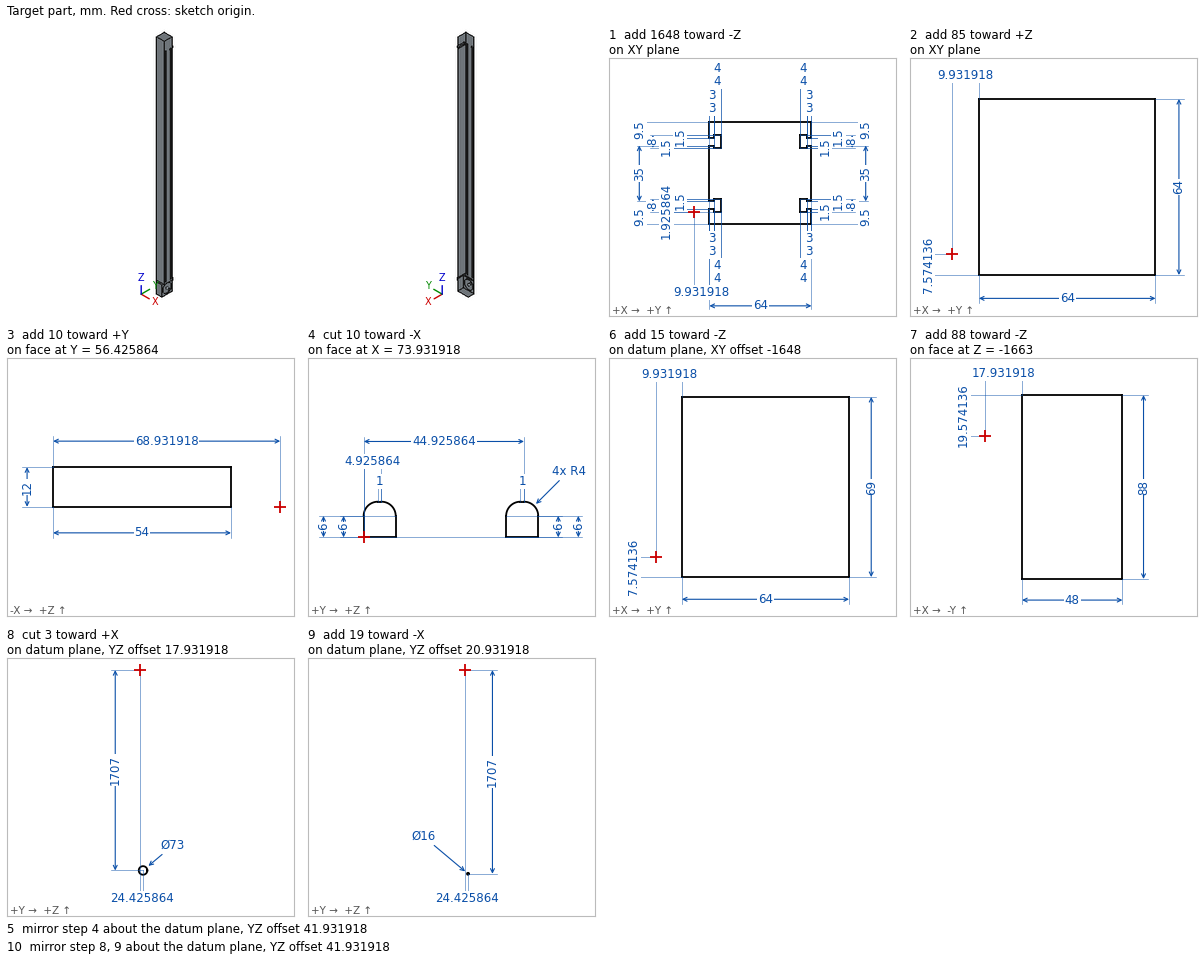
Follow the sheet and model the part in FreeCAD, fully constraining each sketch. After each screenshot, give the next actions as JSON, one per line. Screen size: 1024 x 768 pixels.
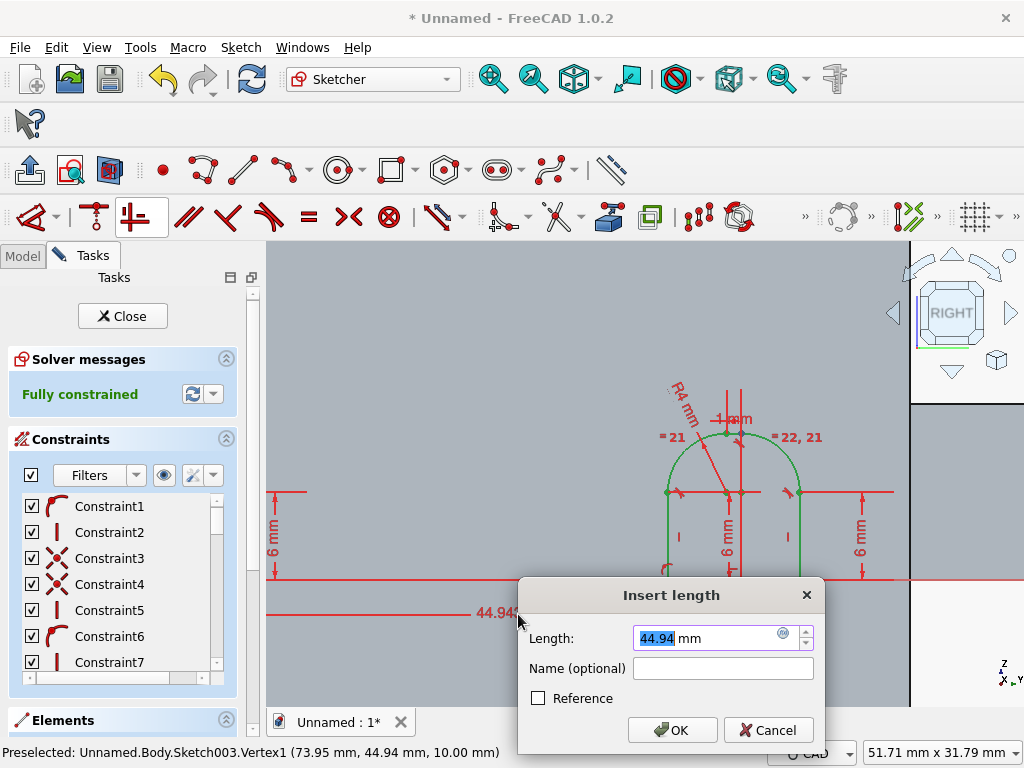
{"action": "type", "text": "44.925864"}
{"action": "key", "text": "Return"}
{"action": "key", "text": "Escape"}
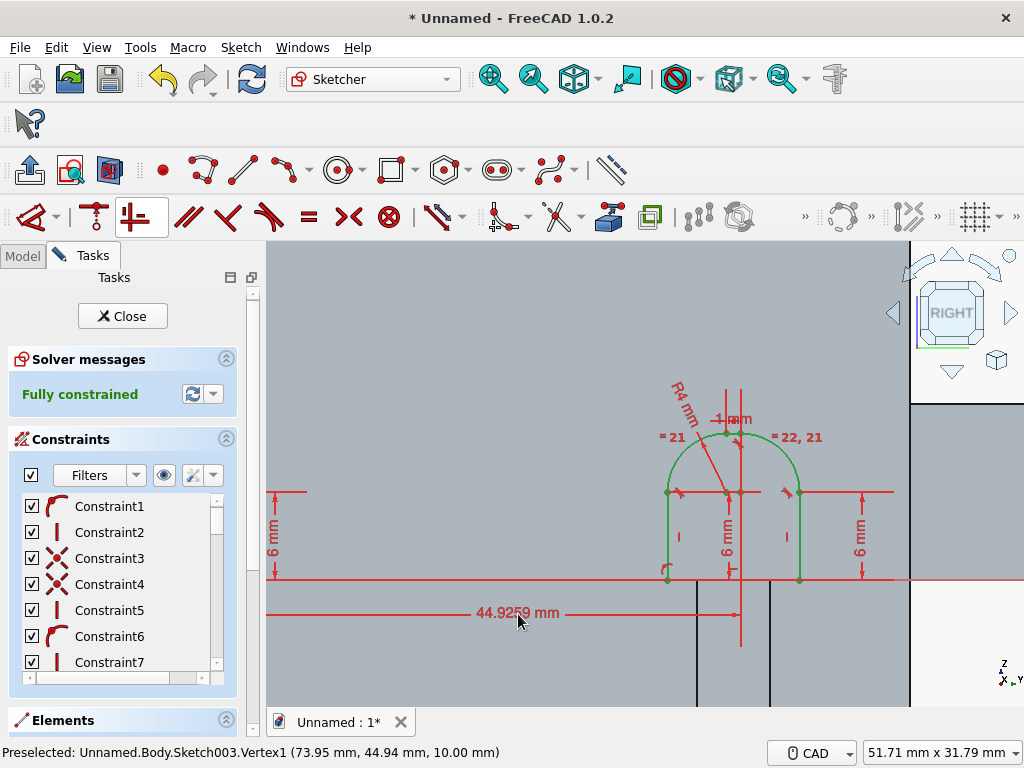
{"action": "left_click", "coordinate": [123, 316]}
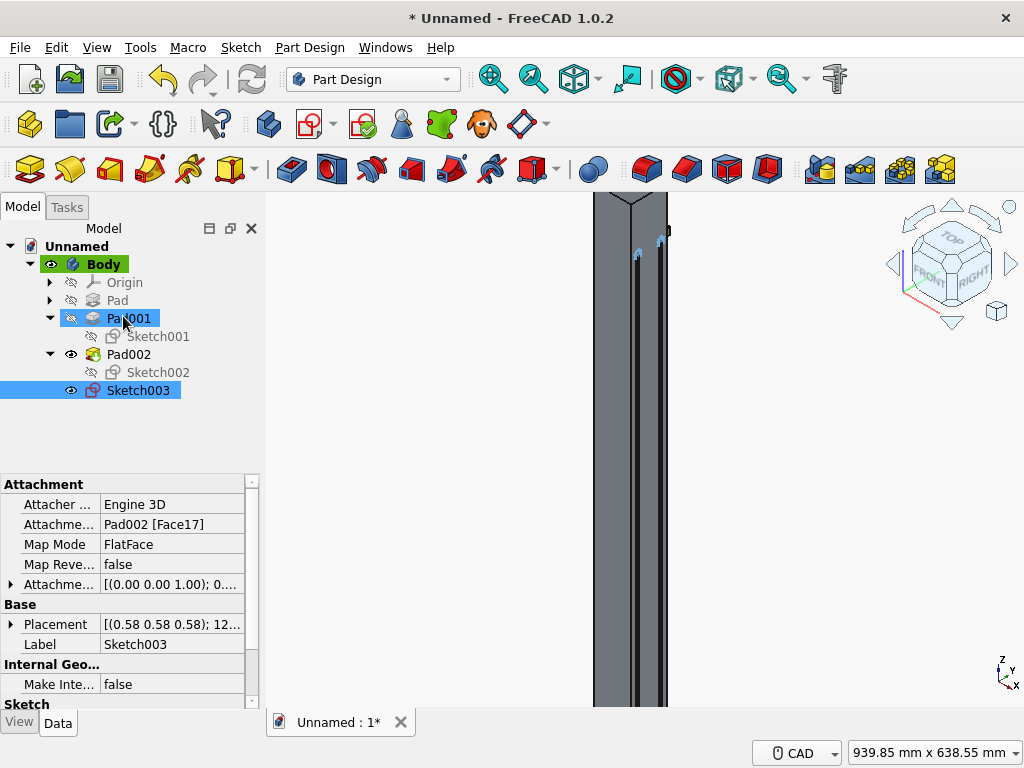
{"action": "left_click", "coordinate": [292, 170]}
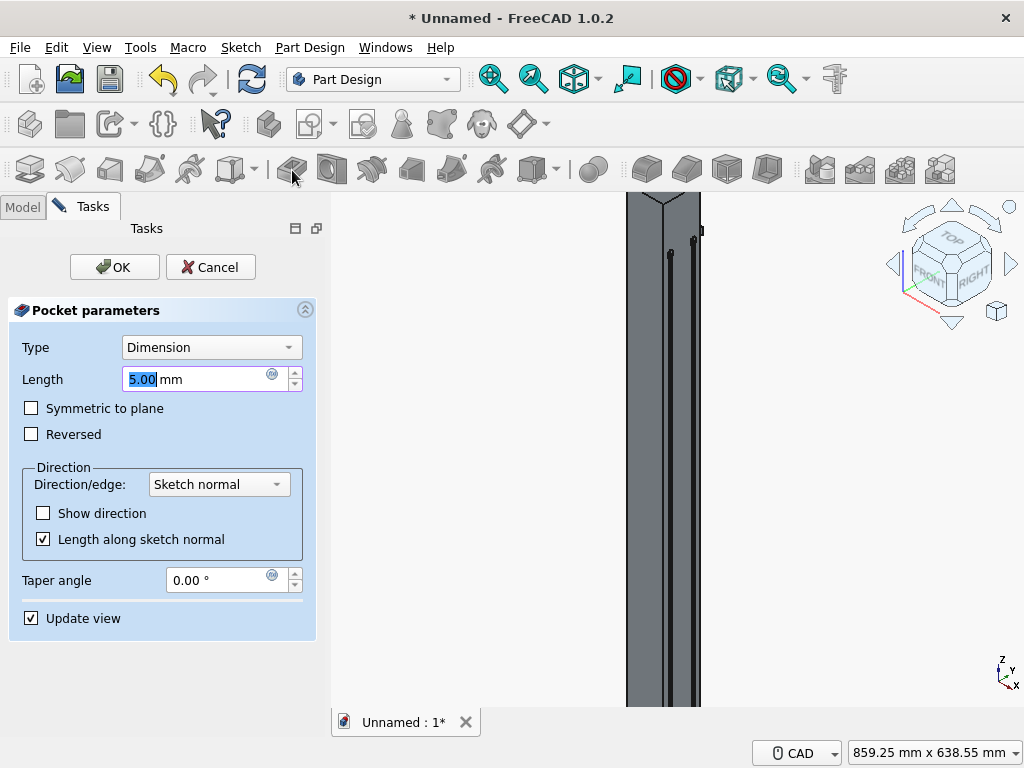
{"action": "type", "text": "10"}
{"action": "key", "text": "Tab"}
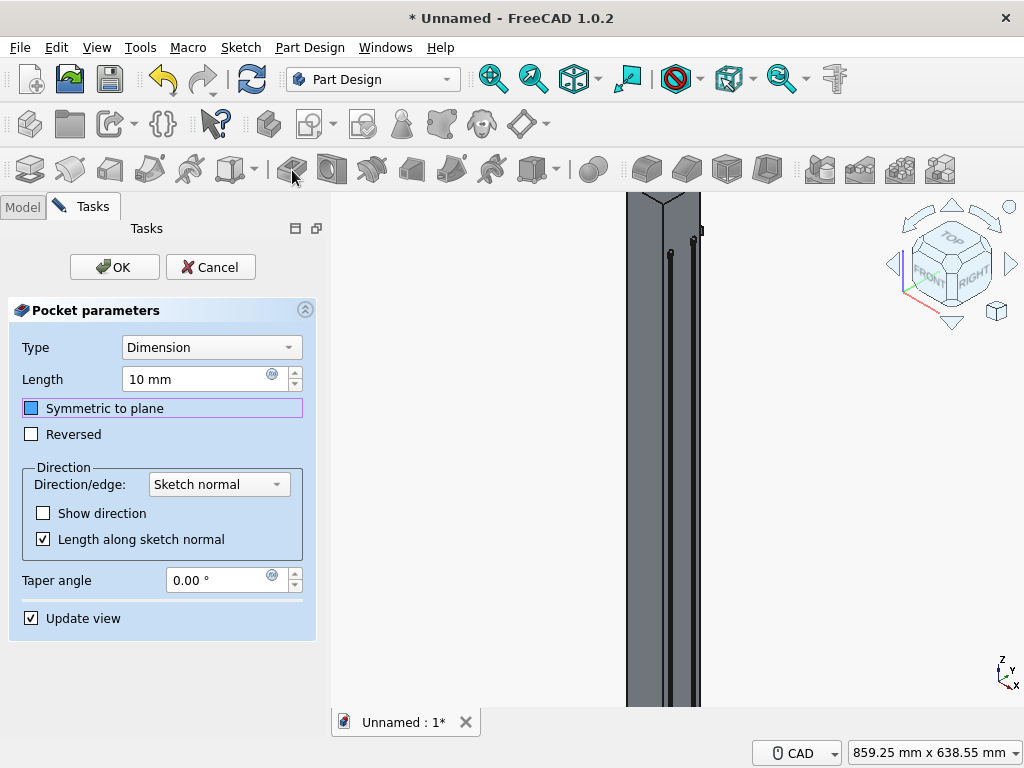
{"action": "left_click", "coordinate": [115, 267]}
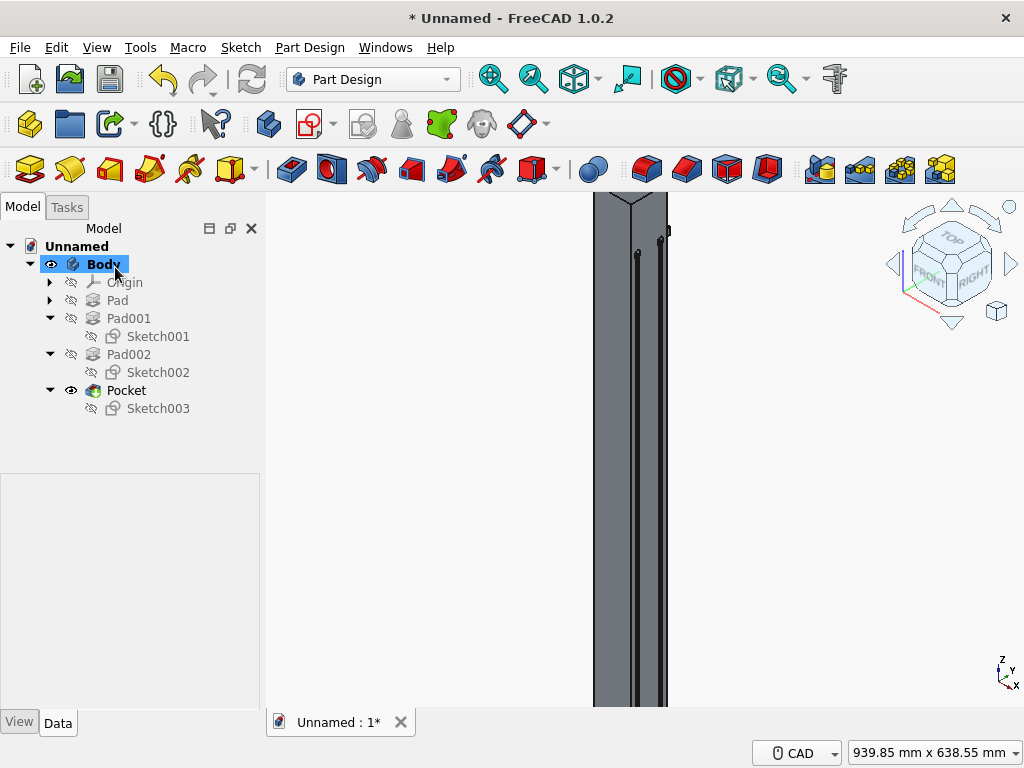
{"action": "left_click", "coordinate": [494, 80]}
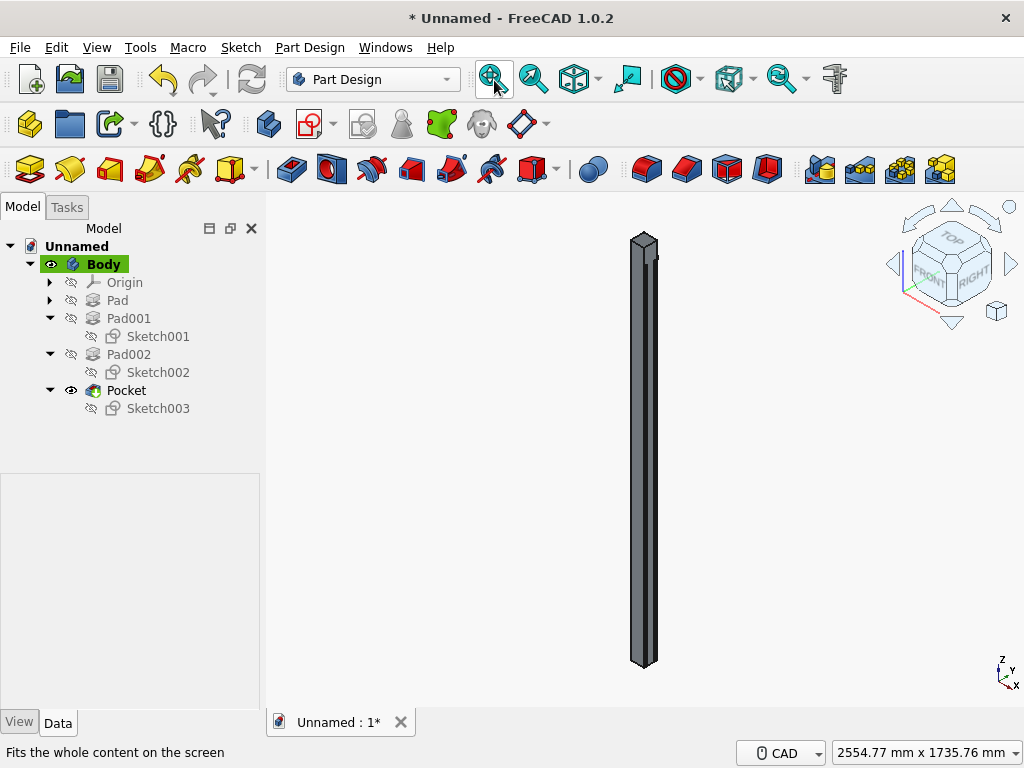
{"action": "left_click", "coordinate": [50, 282]}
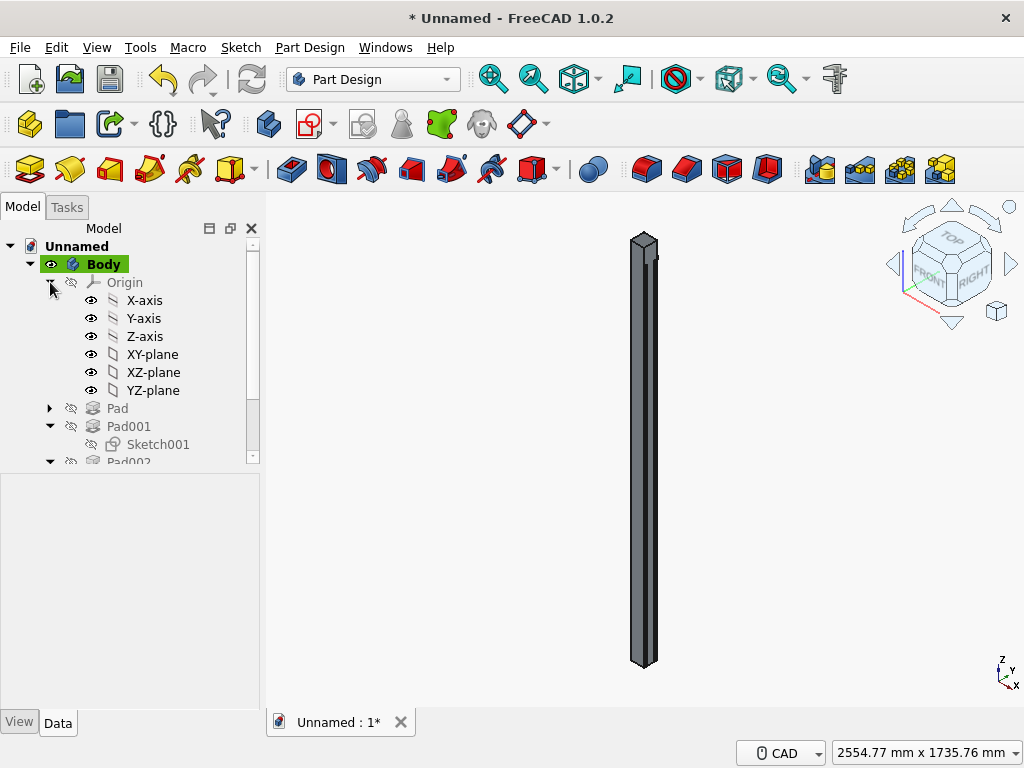
{"action": "left_click", "coordinate": [136, 390]}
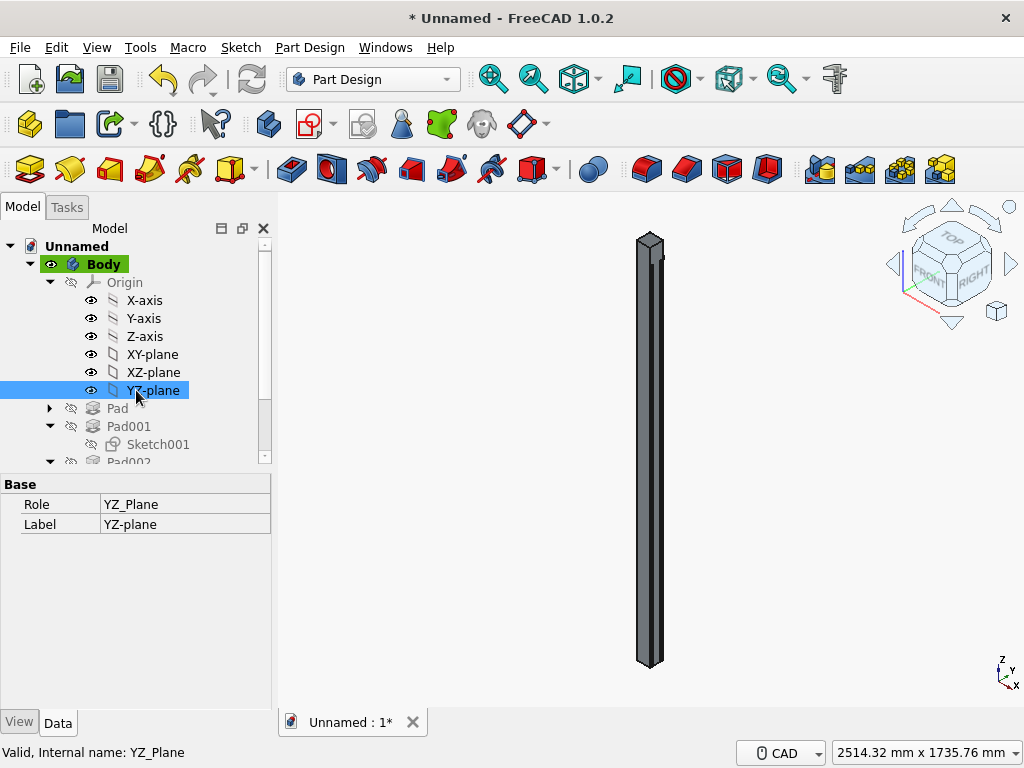
{"action": "left_click", "coordinate": [522, 124]}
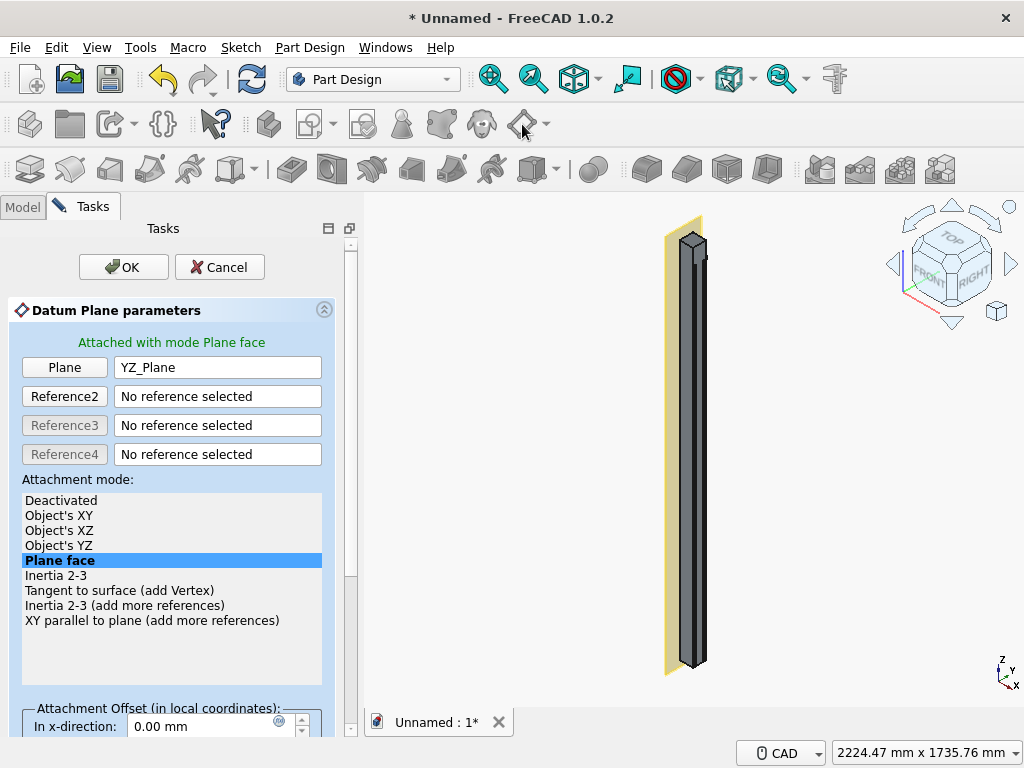
{"action": "scroll", "coordinate": [351, 487], "scroll_direction": "down", "scroll_amount": 3}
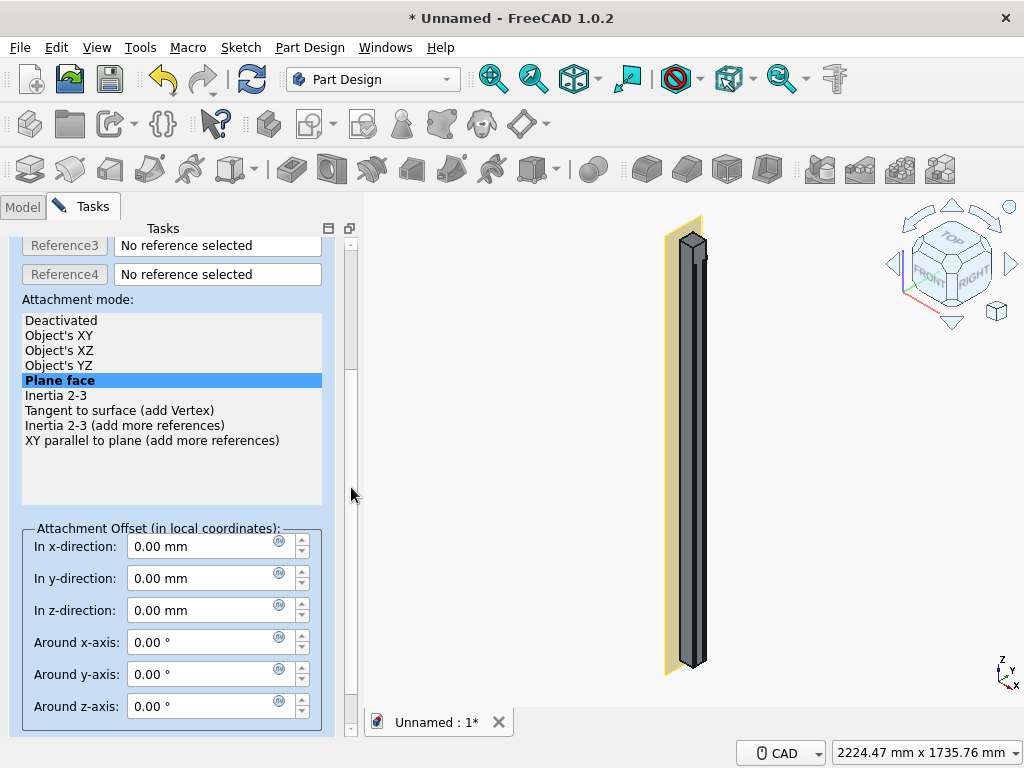
{"action": "triple_click", "coordinate": [210, 610]}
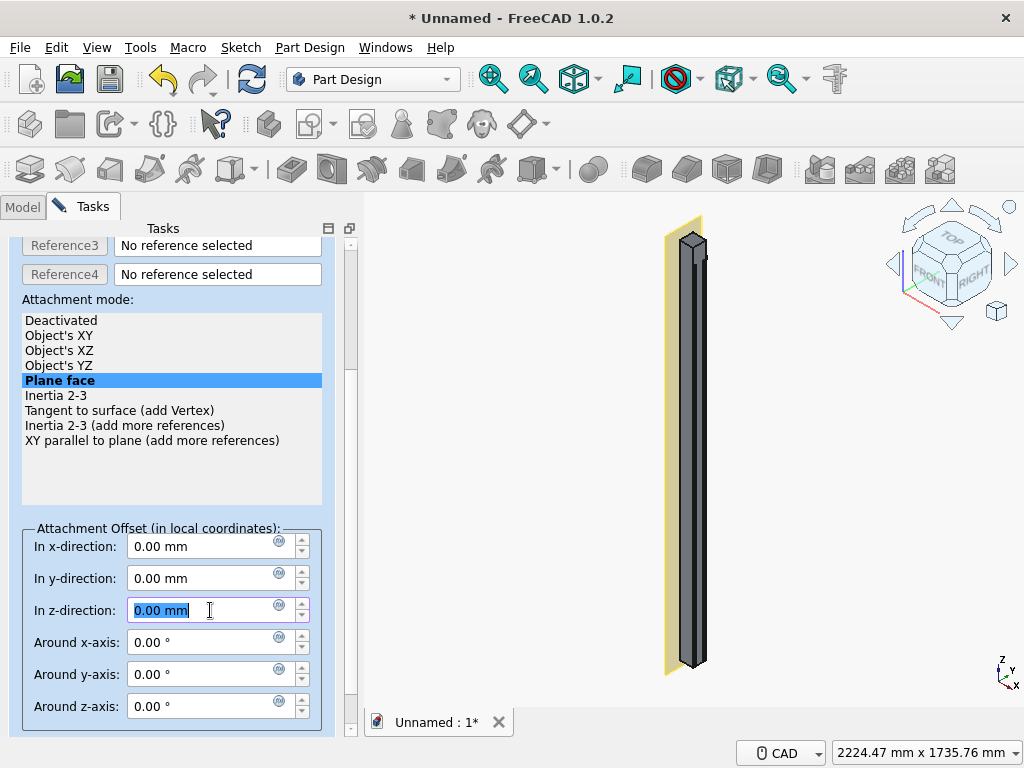
{"action": "type", "text": "41.931918"}
{"action": "key", "text": "Tab"}